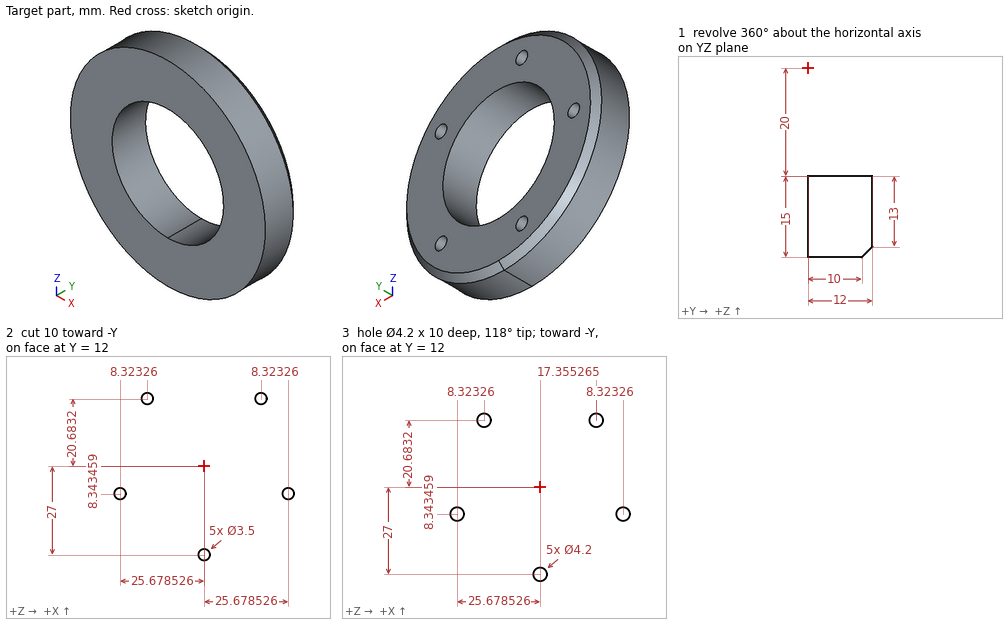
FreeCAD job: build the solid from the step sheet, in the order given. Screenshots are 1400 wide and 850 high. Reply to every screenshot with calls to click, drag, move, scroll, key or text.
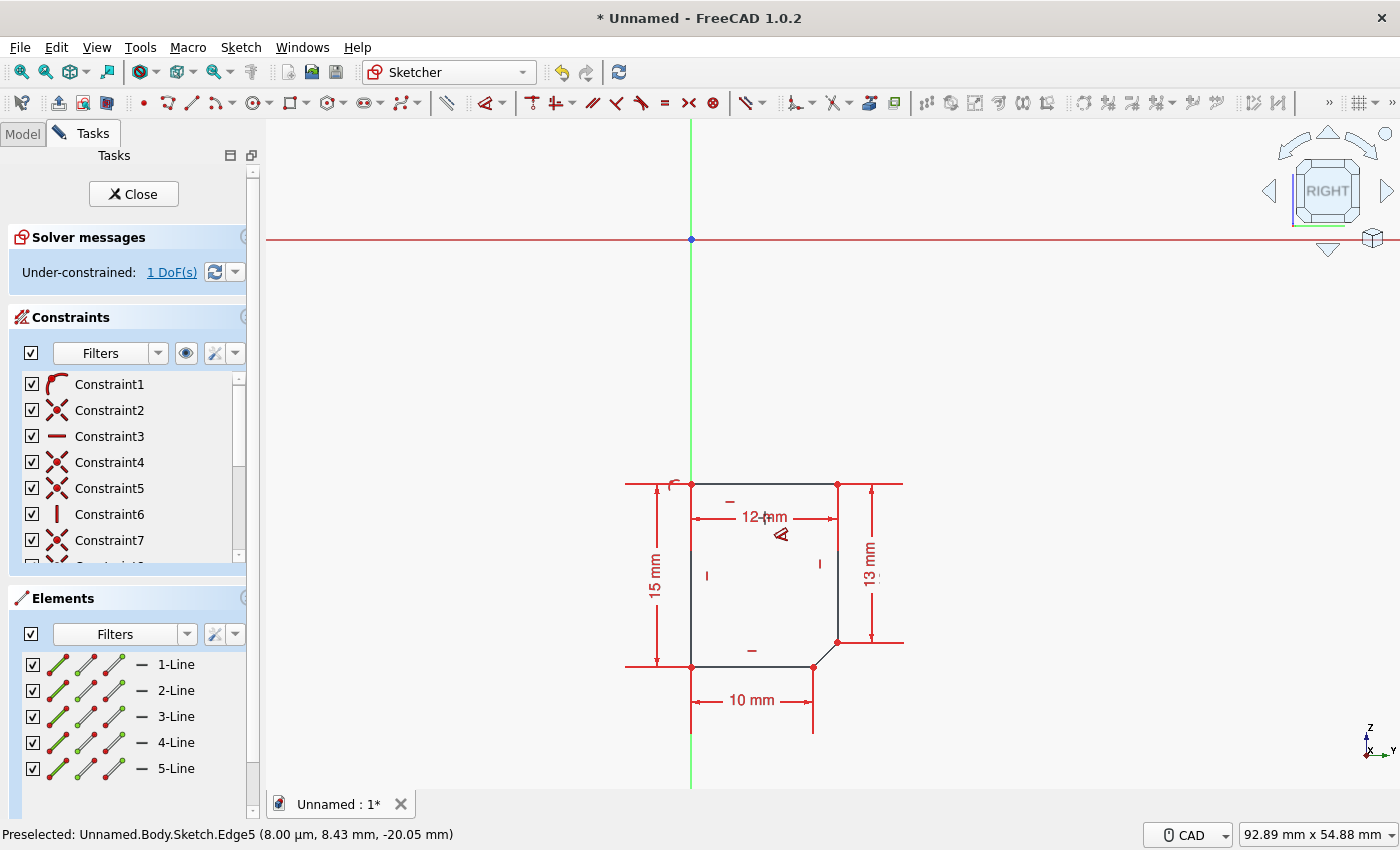
click(691, 484)
click(657, 362)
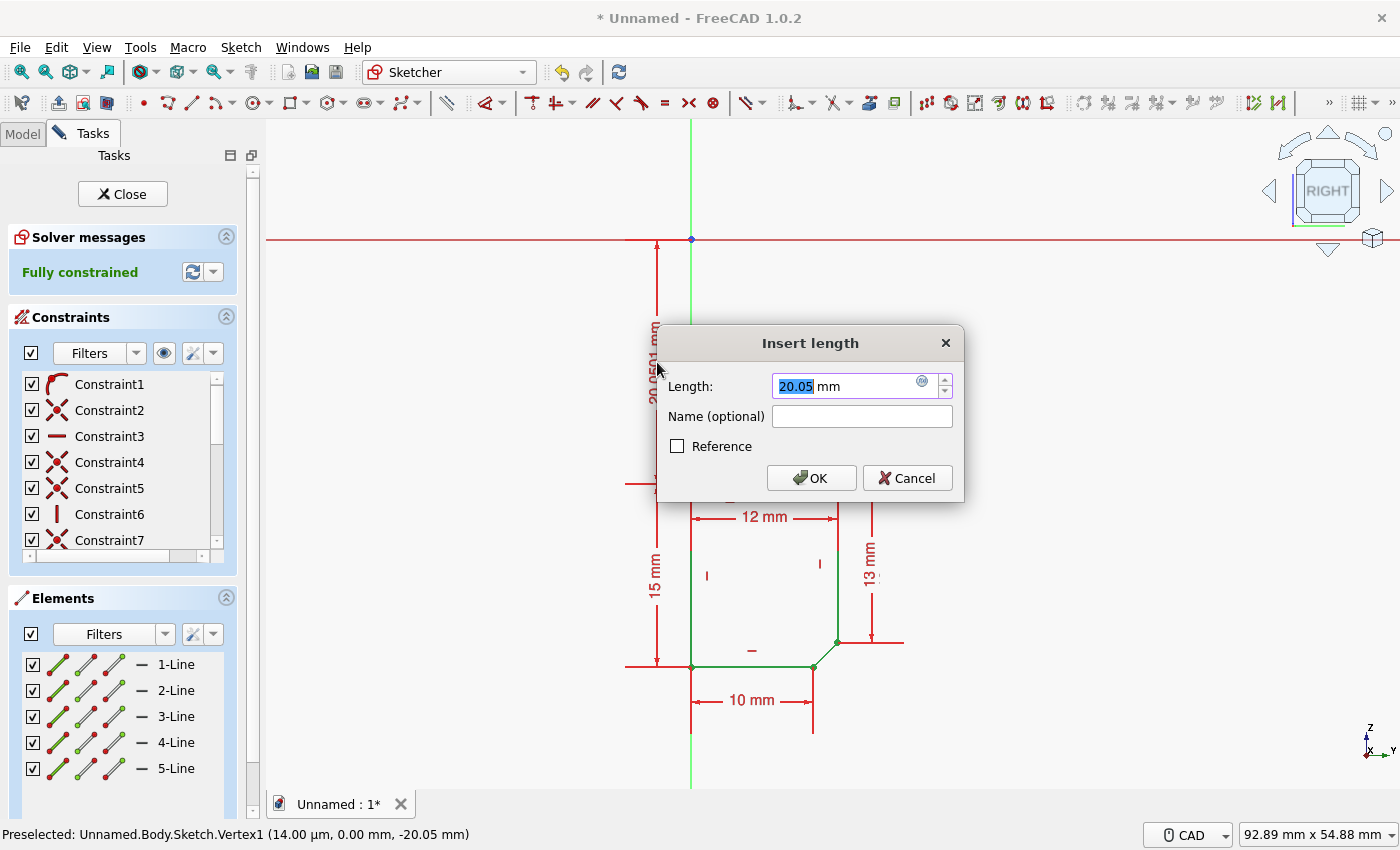
text(20)
key(Return)
key(Escape)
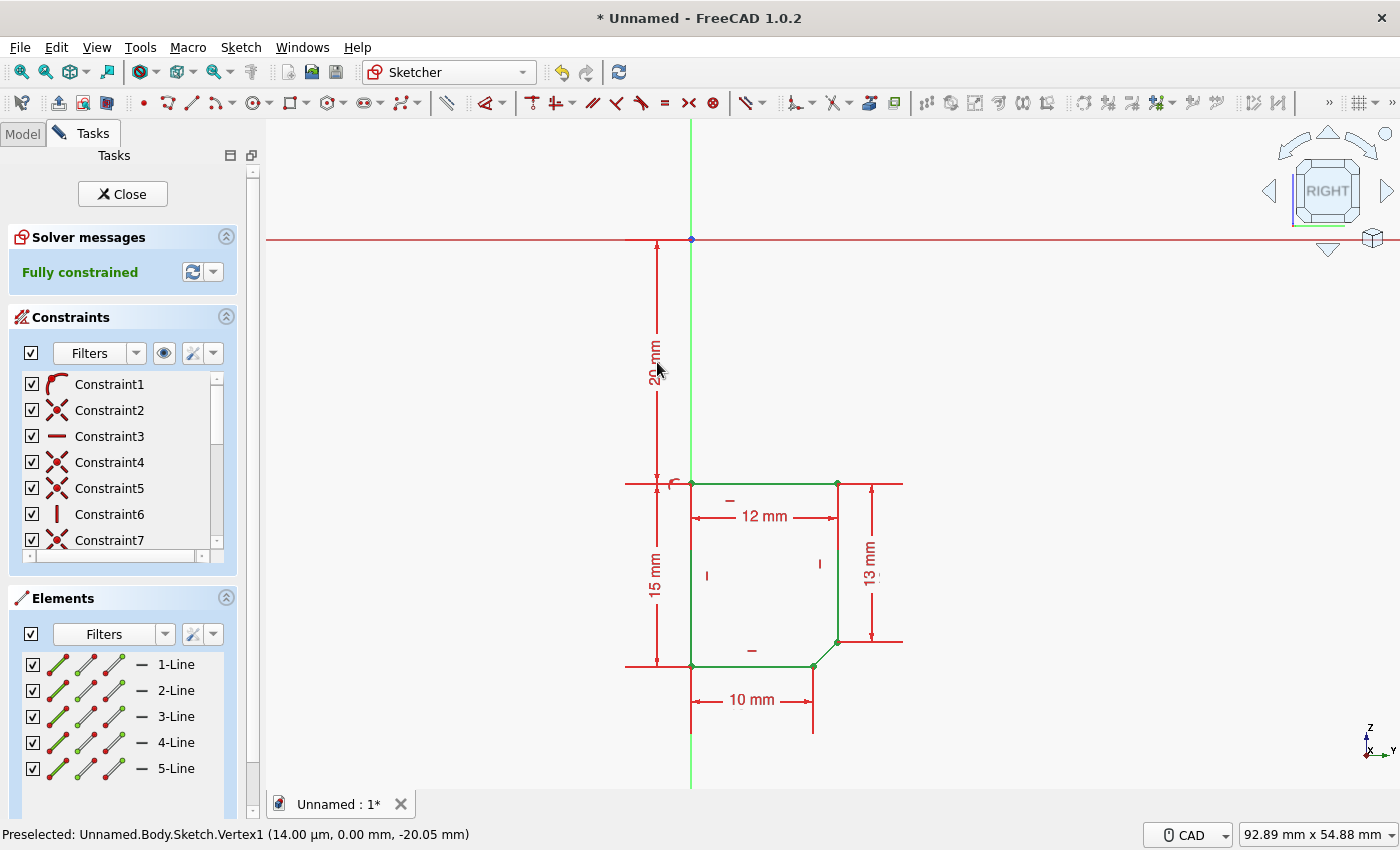
click(123, 194)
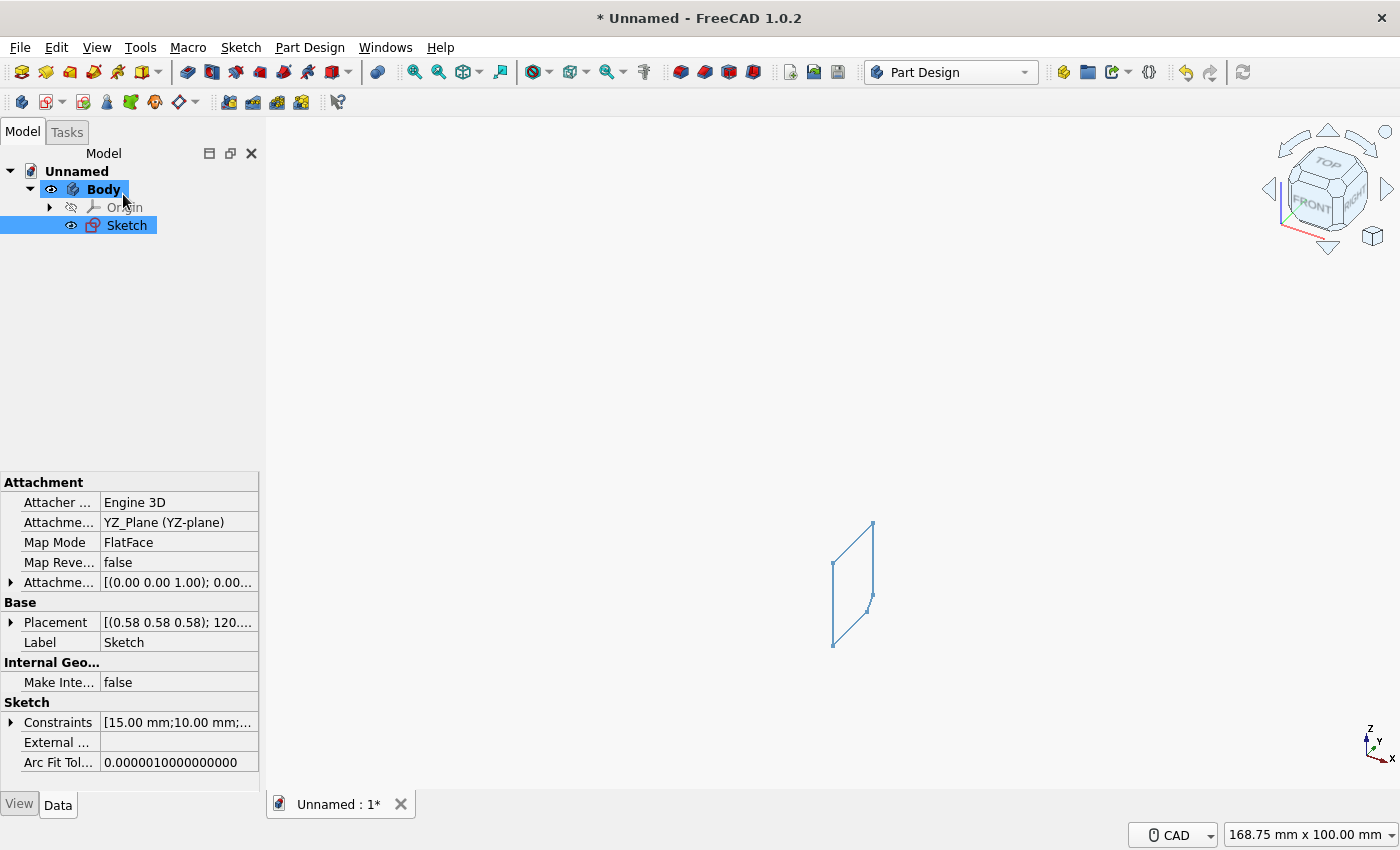
click(46, 72)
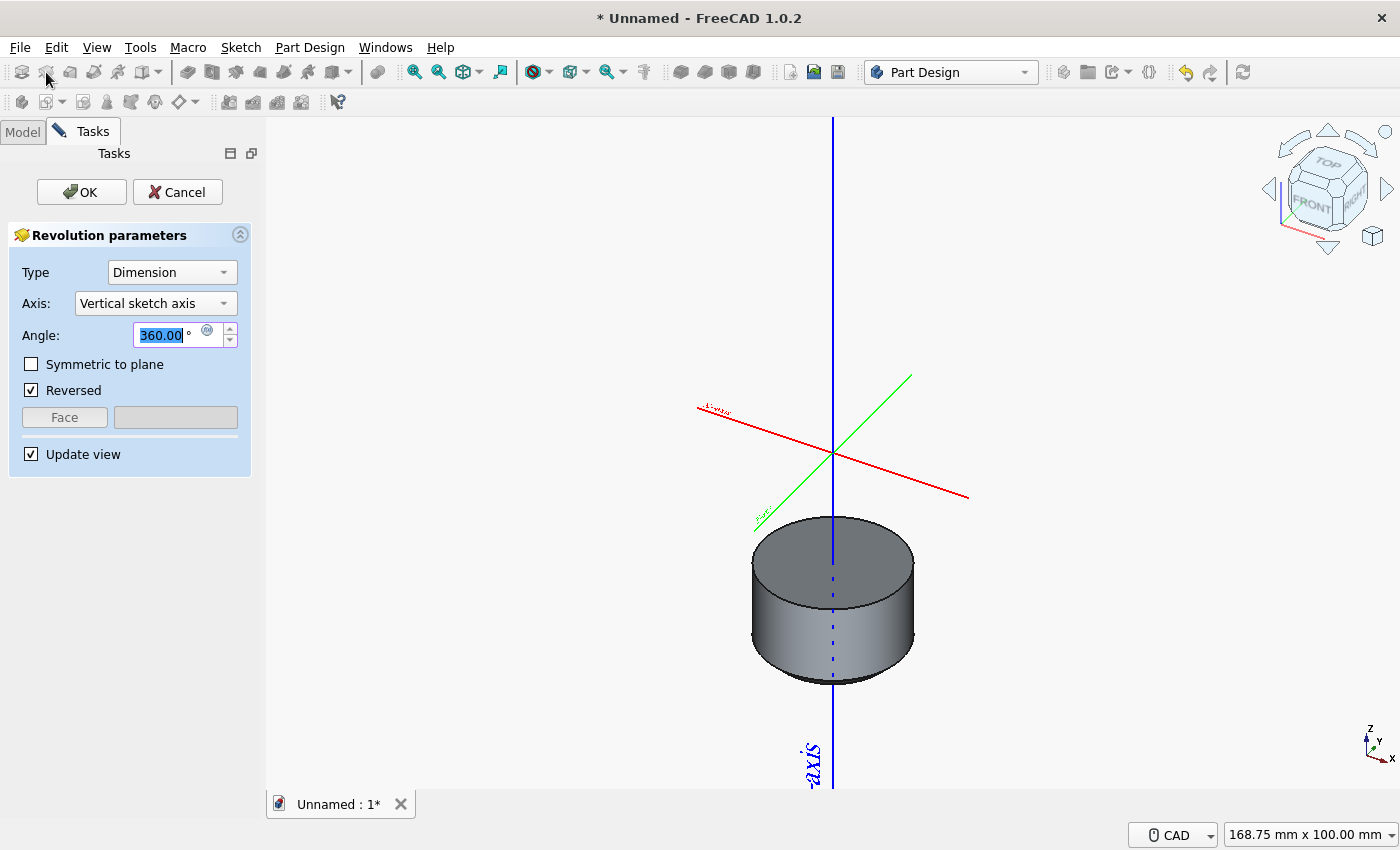
click(156, 304)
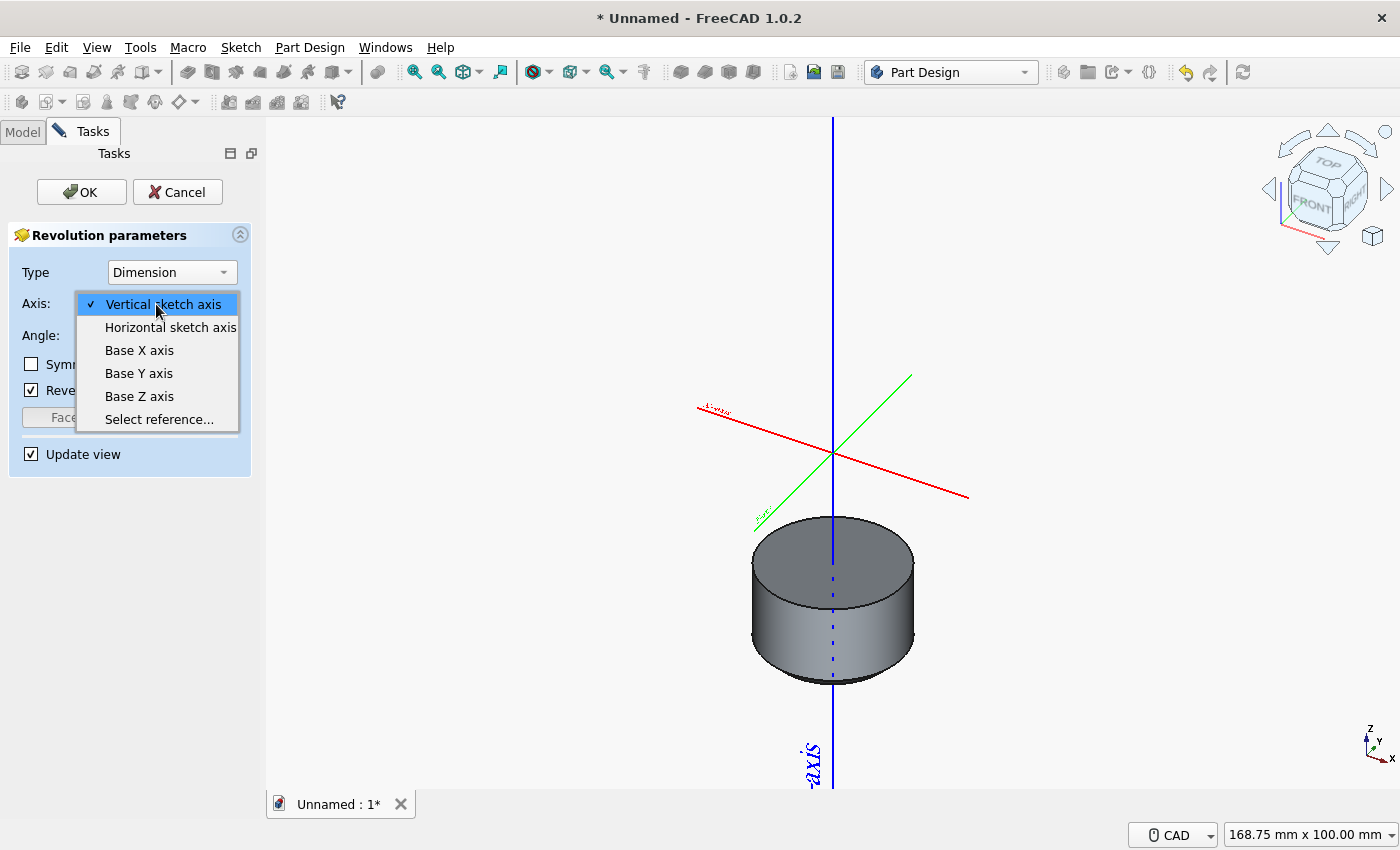
click(156, 328)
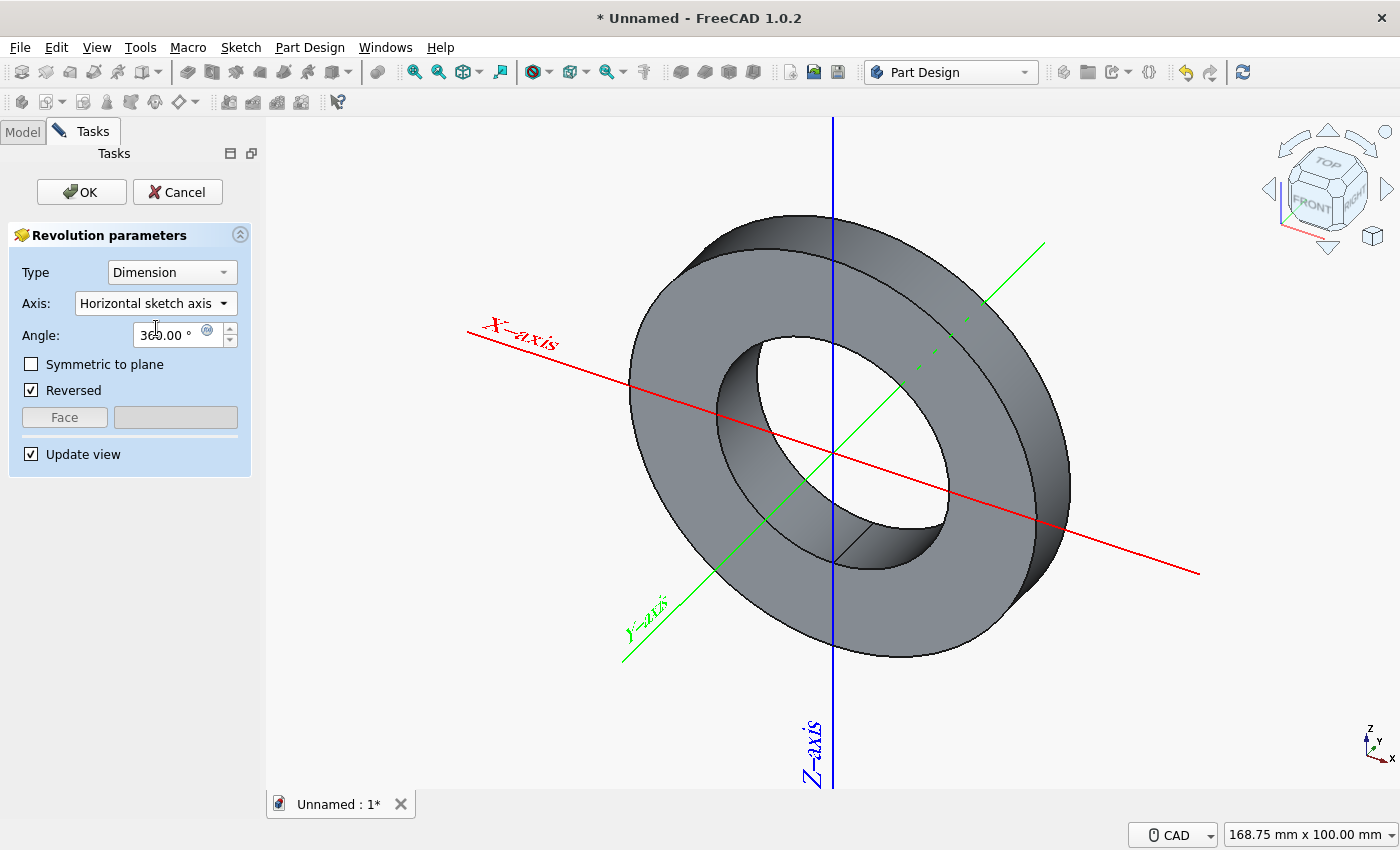
click(82, 192)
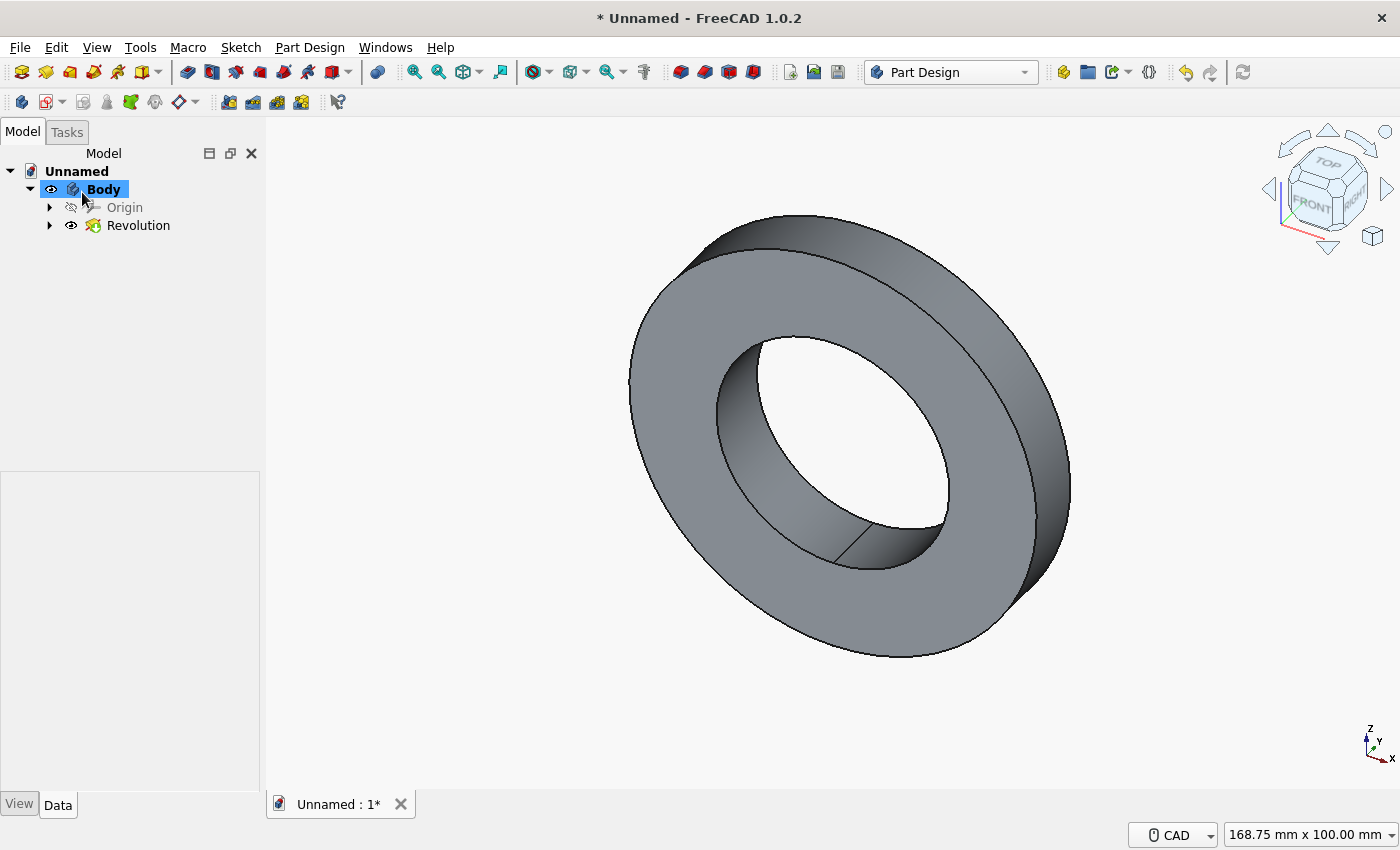
key(4)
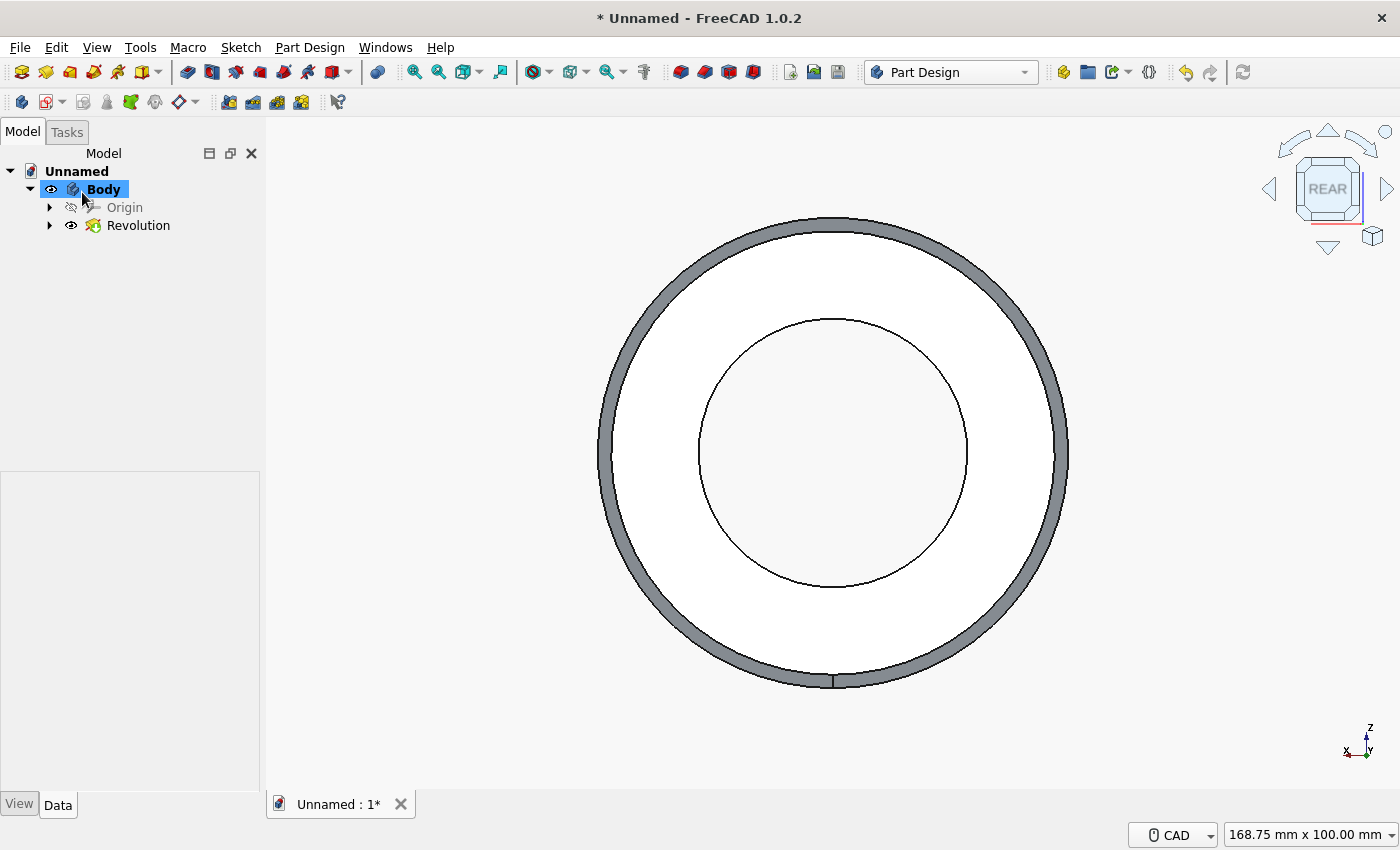
click(960, 325)